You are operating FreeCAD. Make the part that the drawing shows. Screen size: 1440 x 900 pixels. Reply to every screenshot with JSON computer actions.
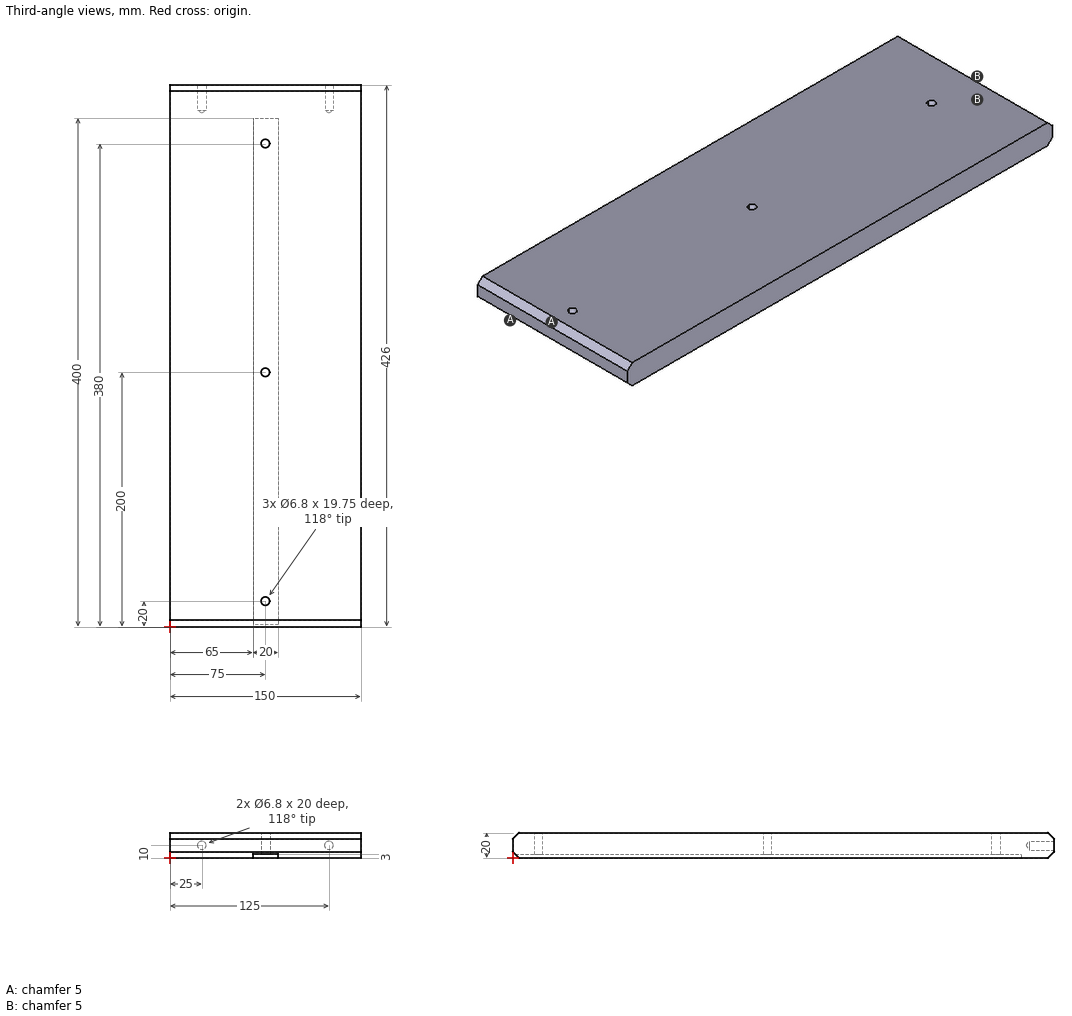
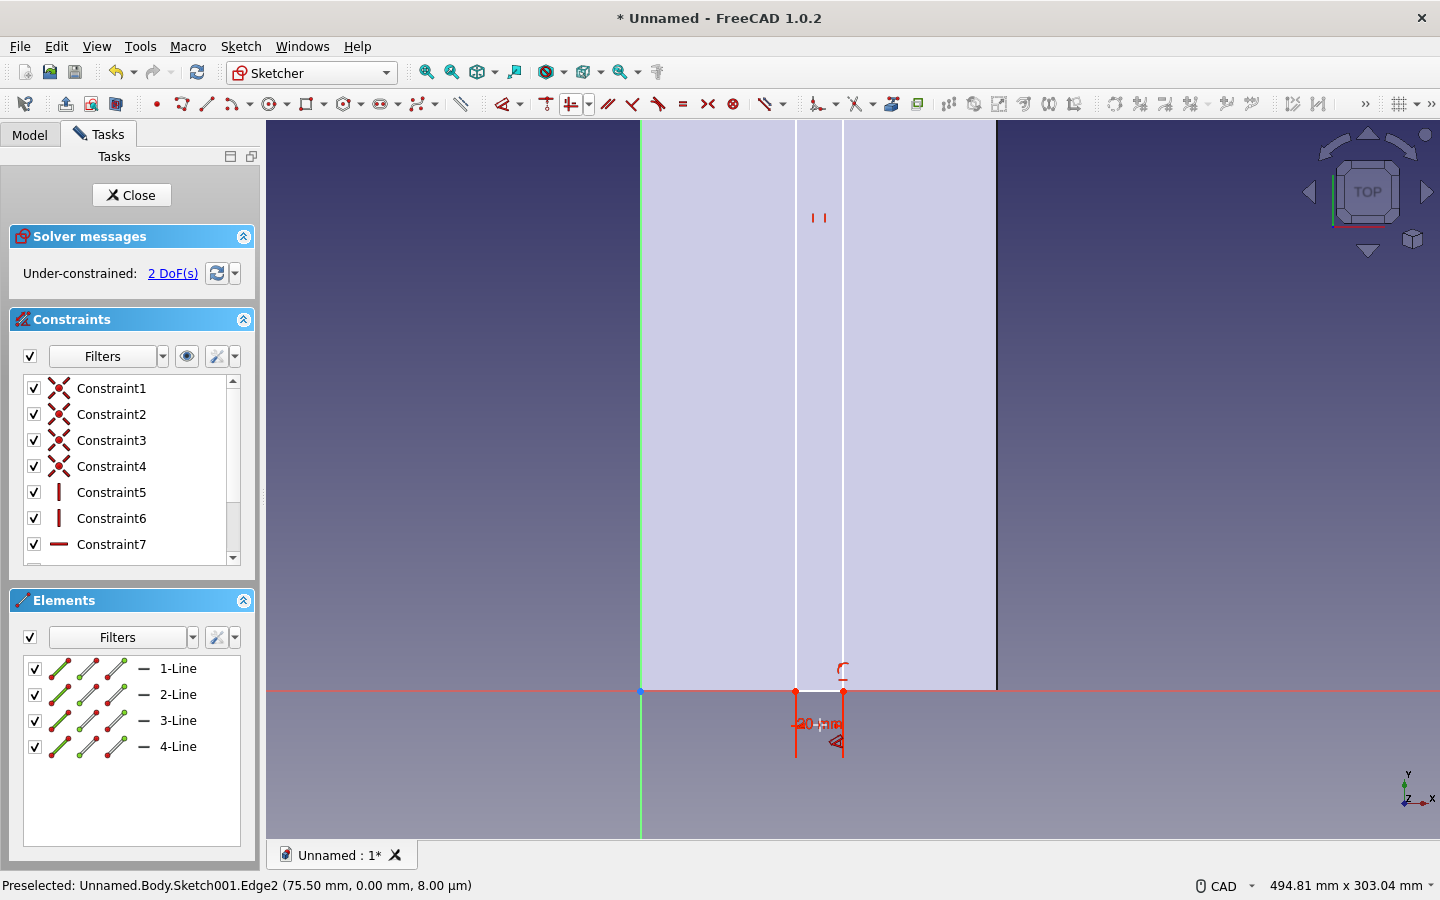
{"action": "left_click", "coordinate": [796, 407]}
{"action": "left_click", "coordinate": [830, 420]}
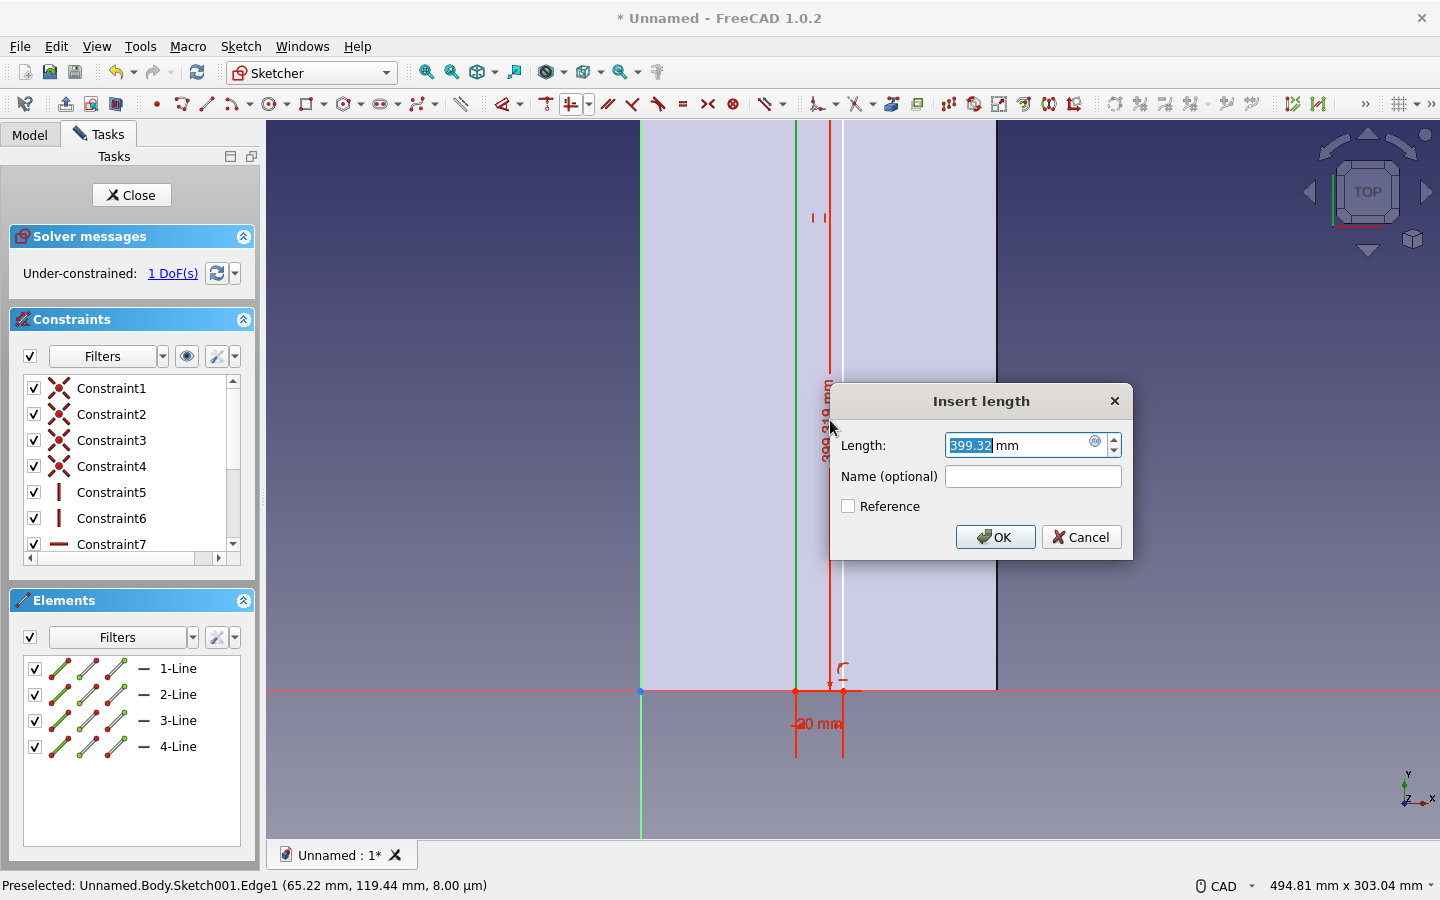
{"action": "type", "text": "400"}
{"action": "key", "text": "Return"}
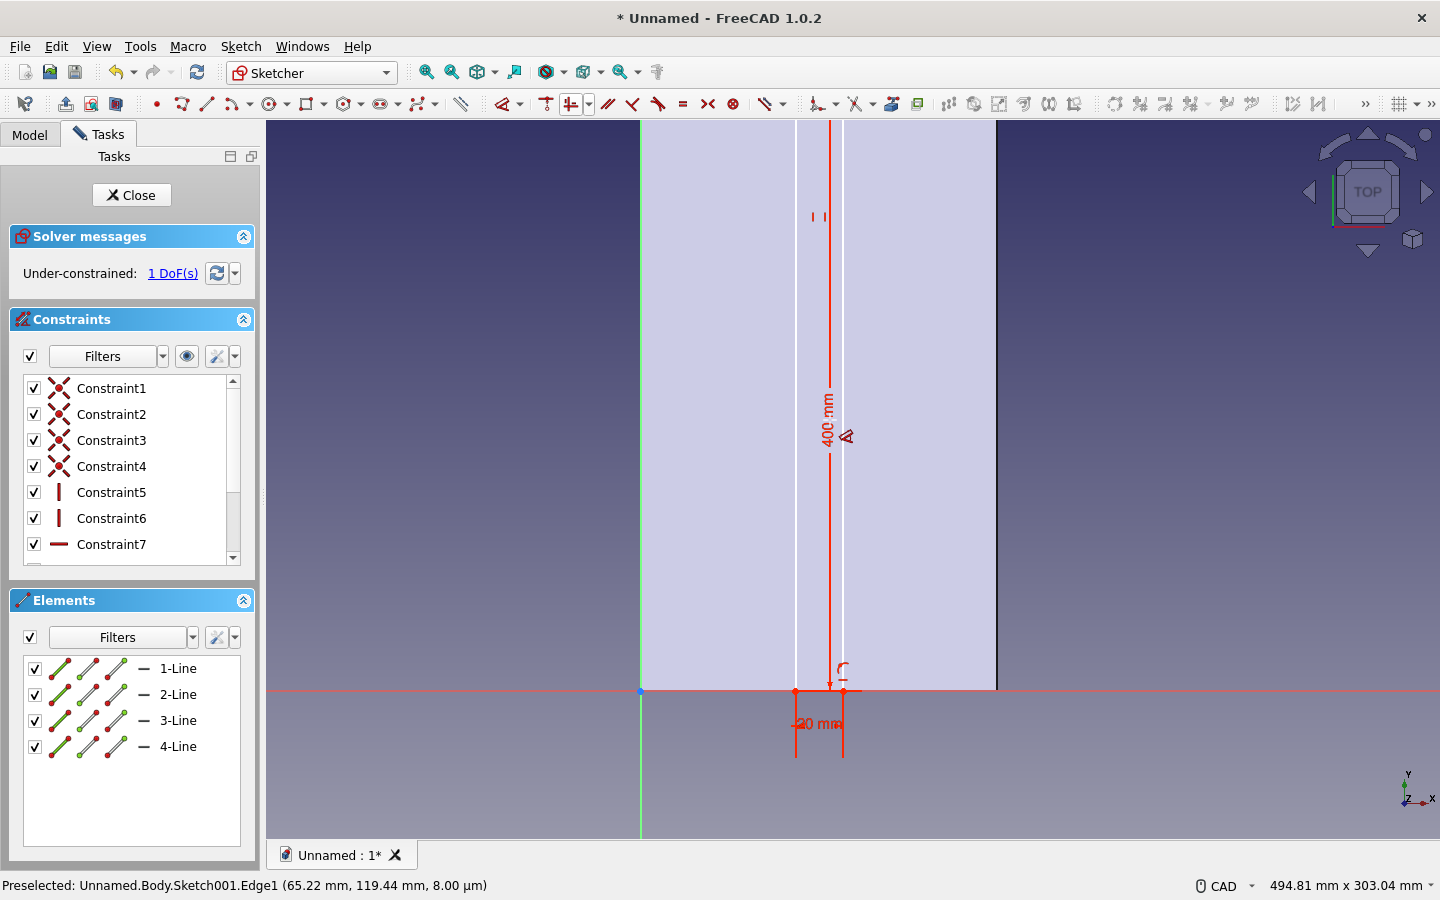
{"action": "scroll", "coordinate": [819, 694], "scroll_direction": "down", "scroll_amount": 4}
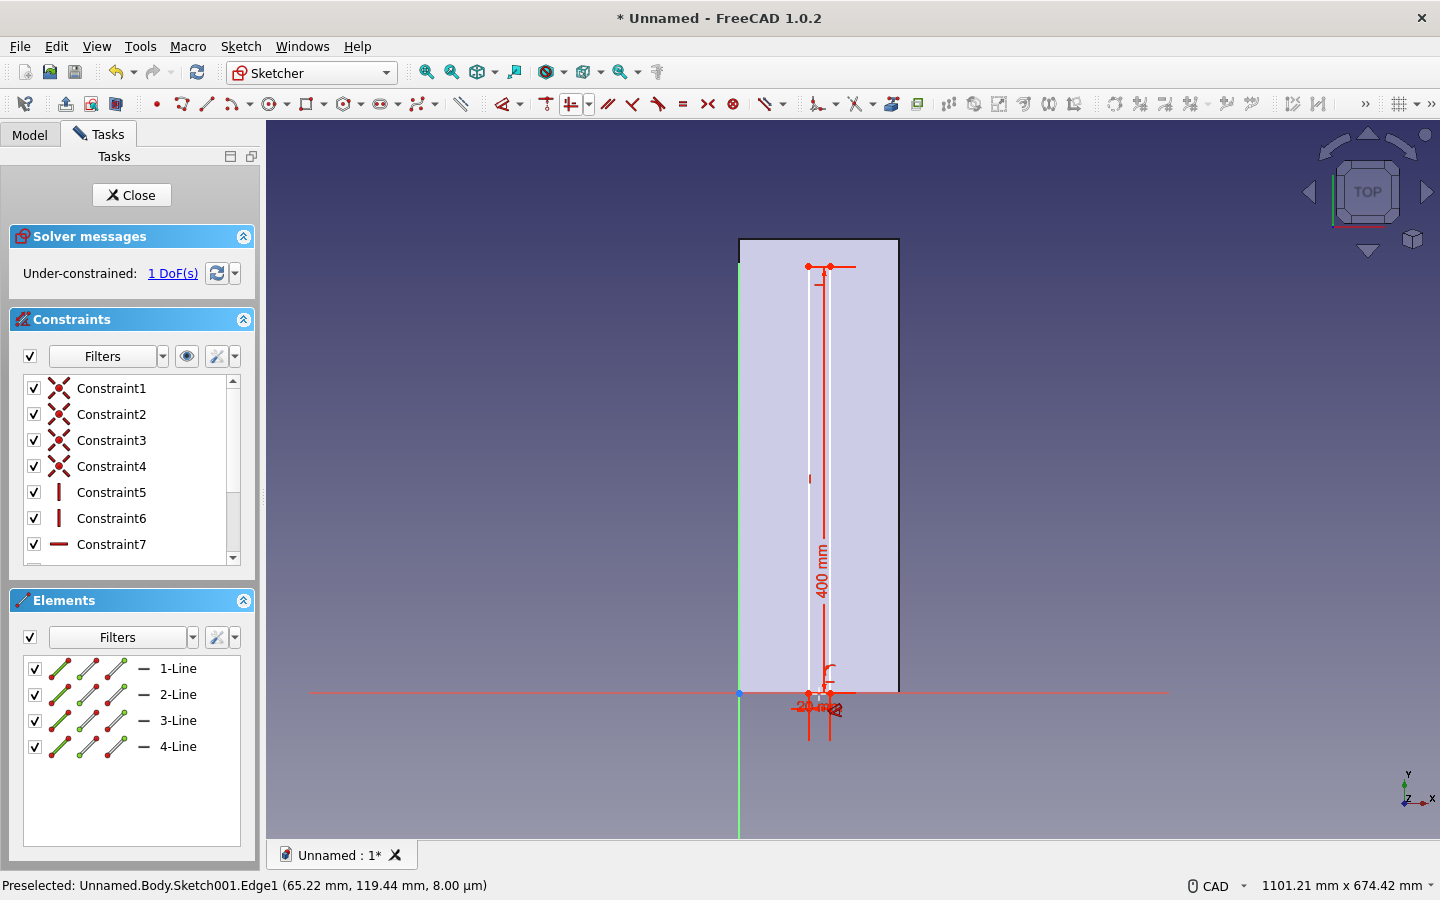
{"action": "left_click", "coordinate": [809, 267]}
{"action": "left_click", "coordinate": [774, 233]}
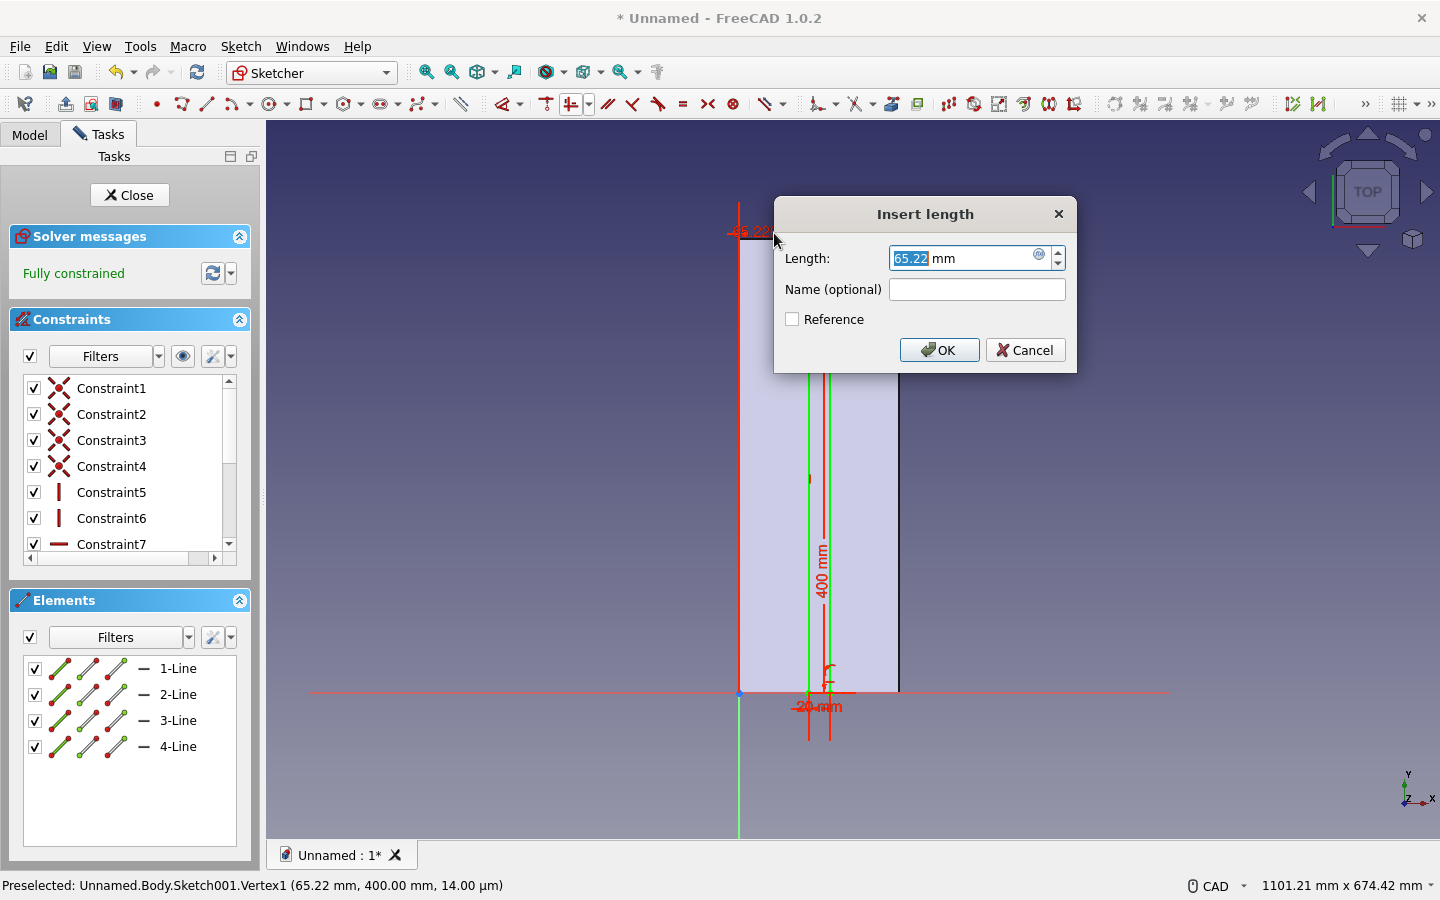
{"action": "type", "text": "65"}
{"action": "key", "text": "Return"}
{"action": "key", "text": "Escape"}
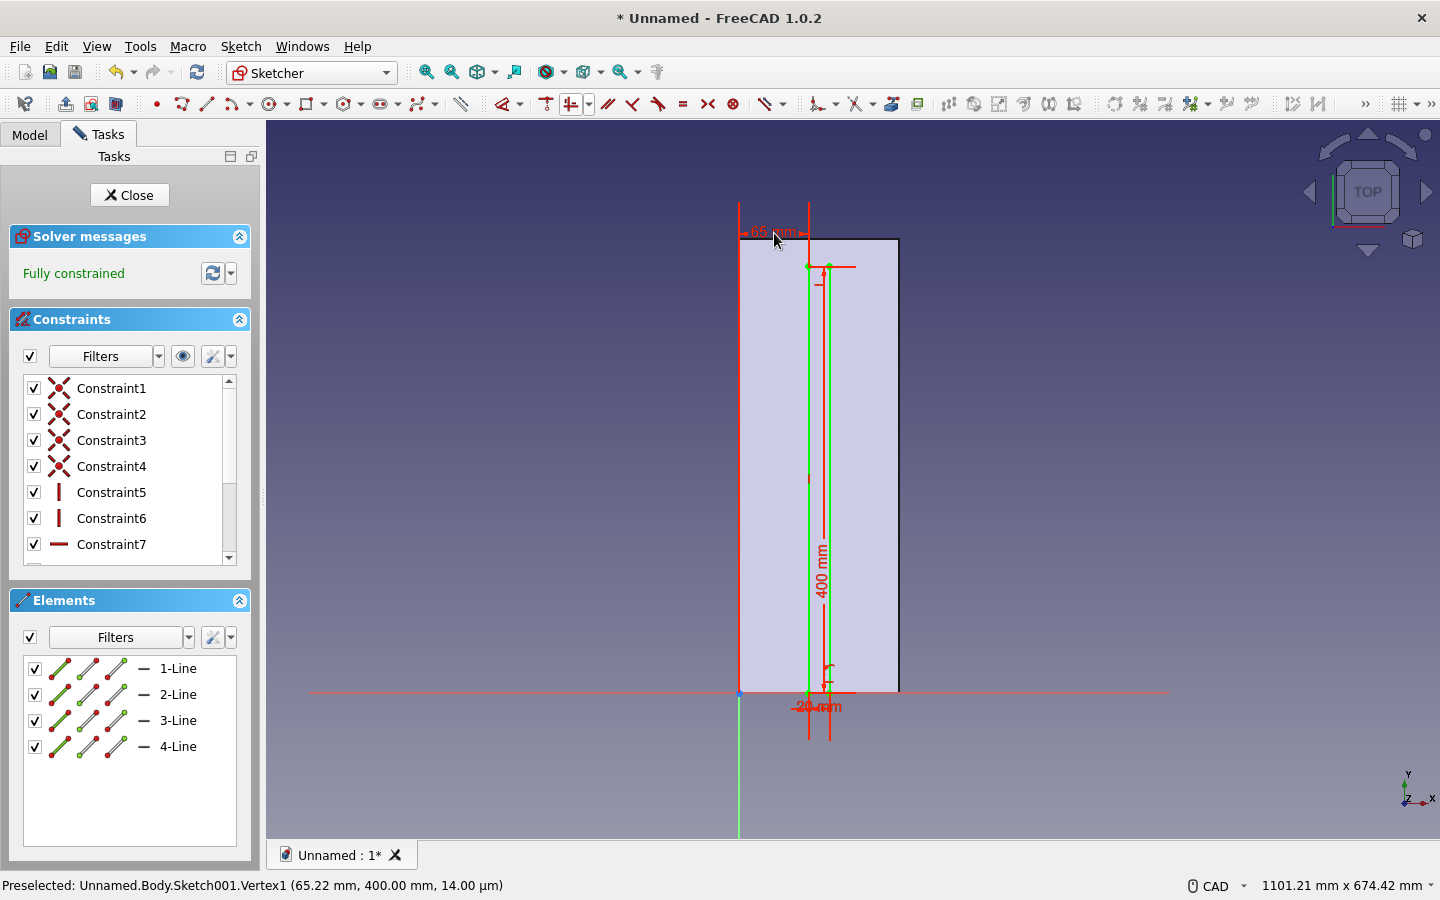
{"action": "left_click", "coordinate": [130, 195]}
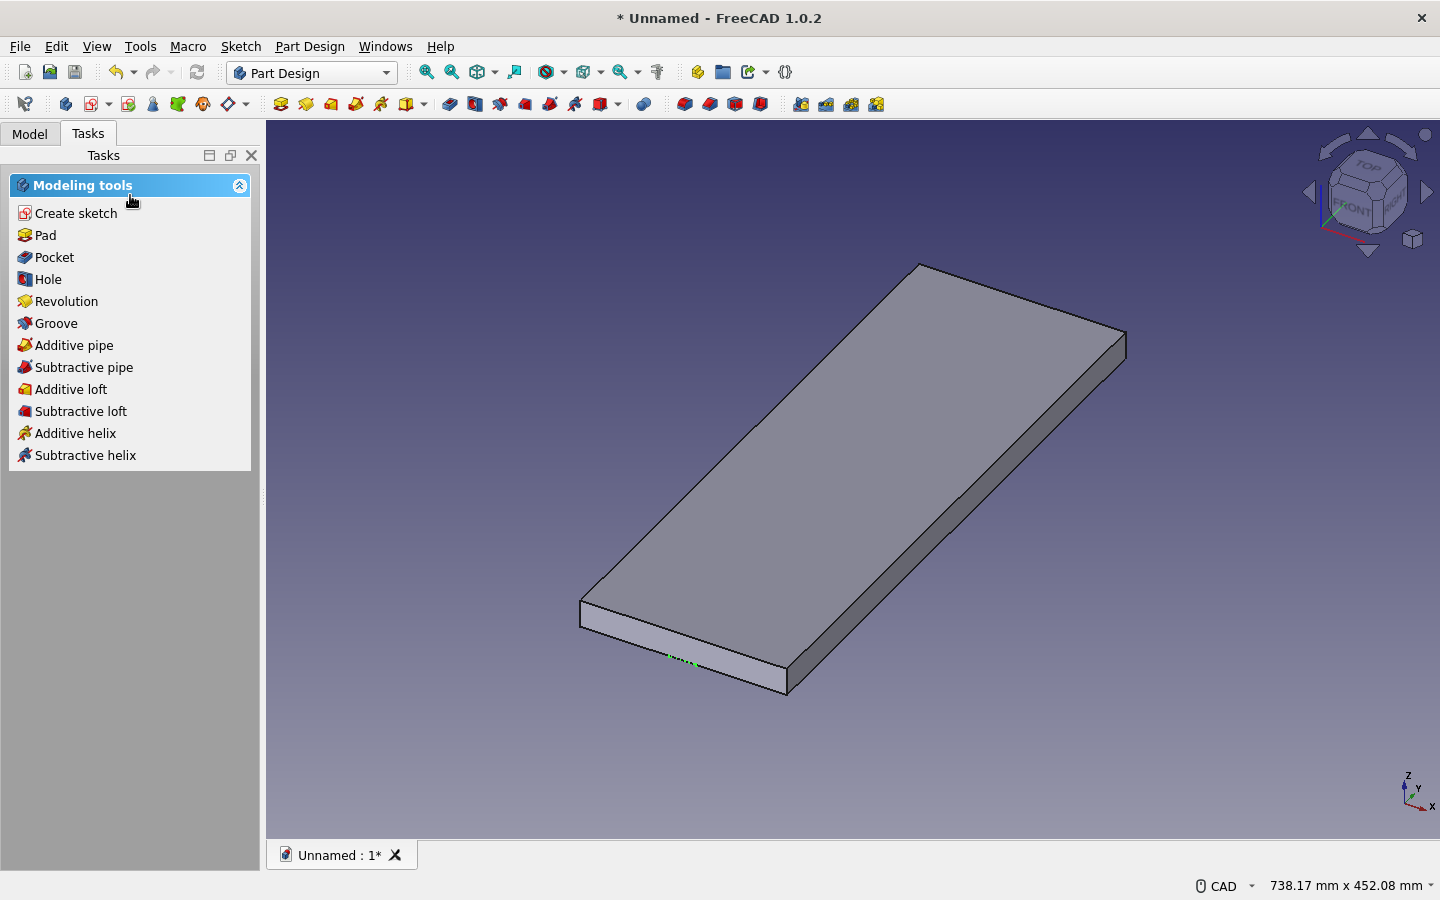
{"action": "left_click", "coordinate": [450, 104]}